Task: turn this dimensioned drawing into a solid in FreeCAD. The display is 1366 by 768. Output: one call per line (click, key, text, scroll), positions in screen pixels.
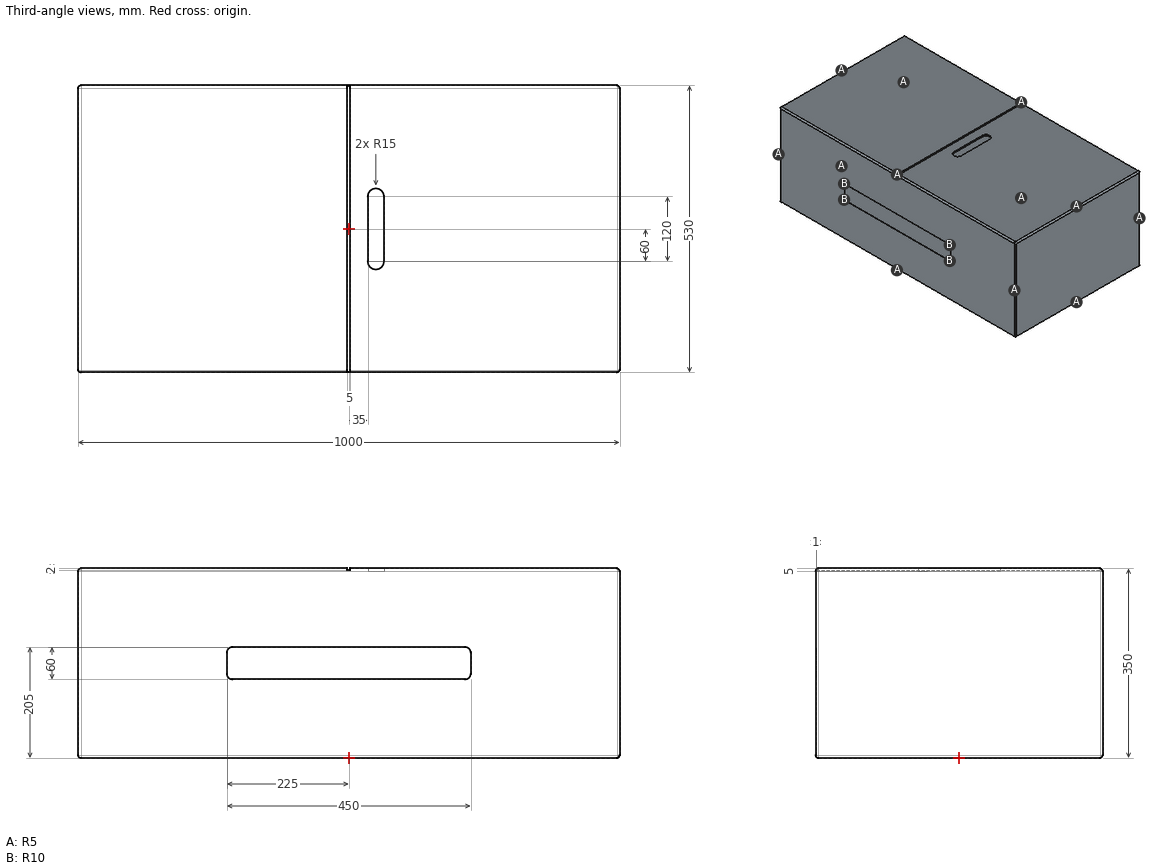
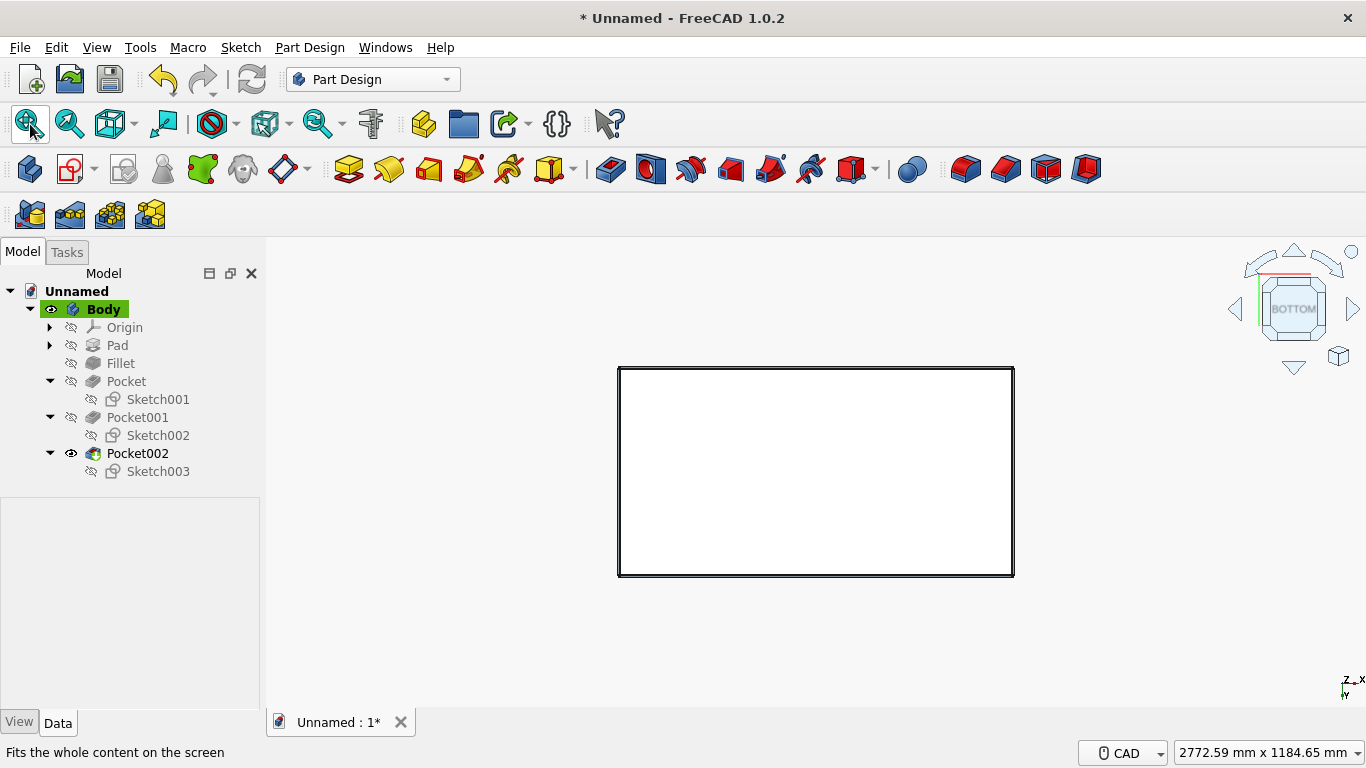
click(30, 124)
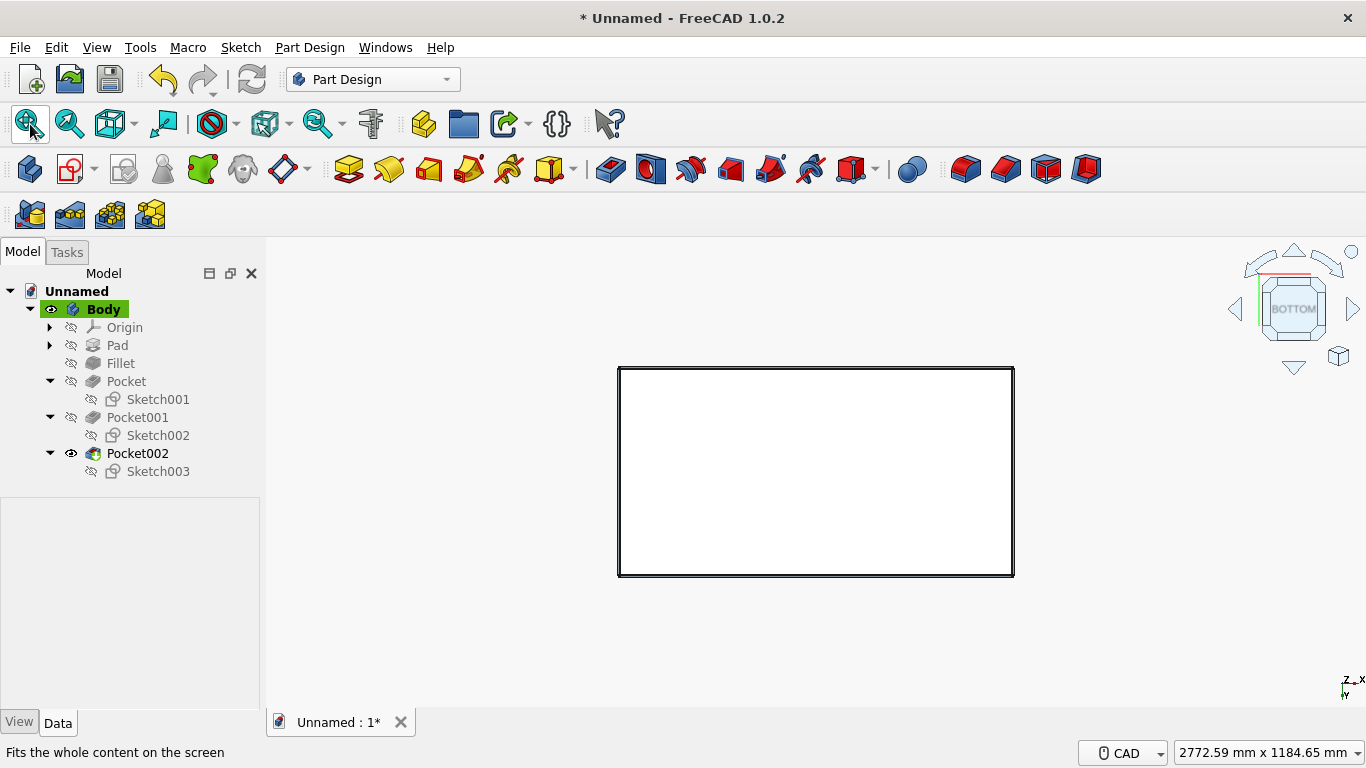
scroll(905, 366, up, 15)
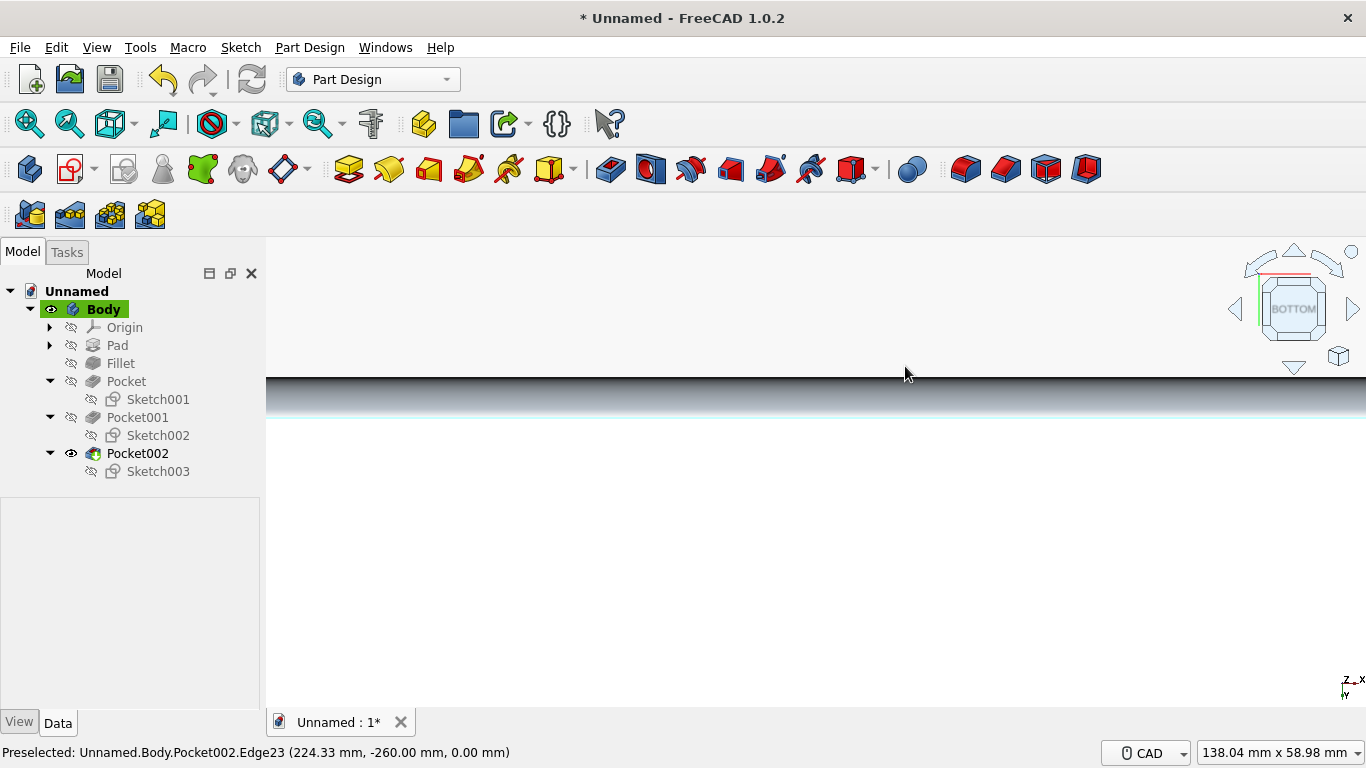
scroll(899, 381, up, 9)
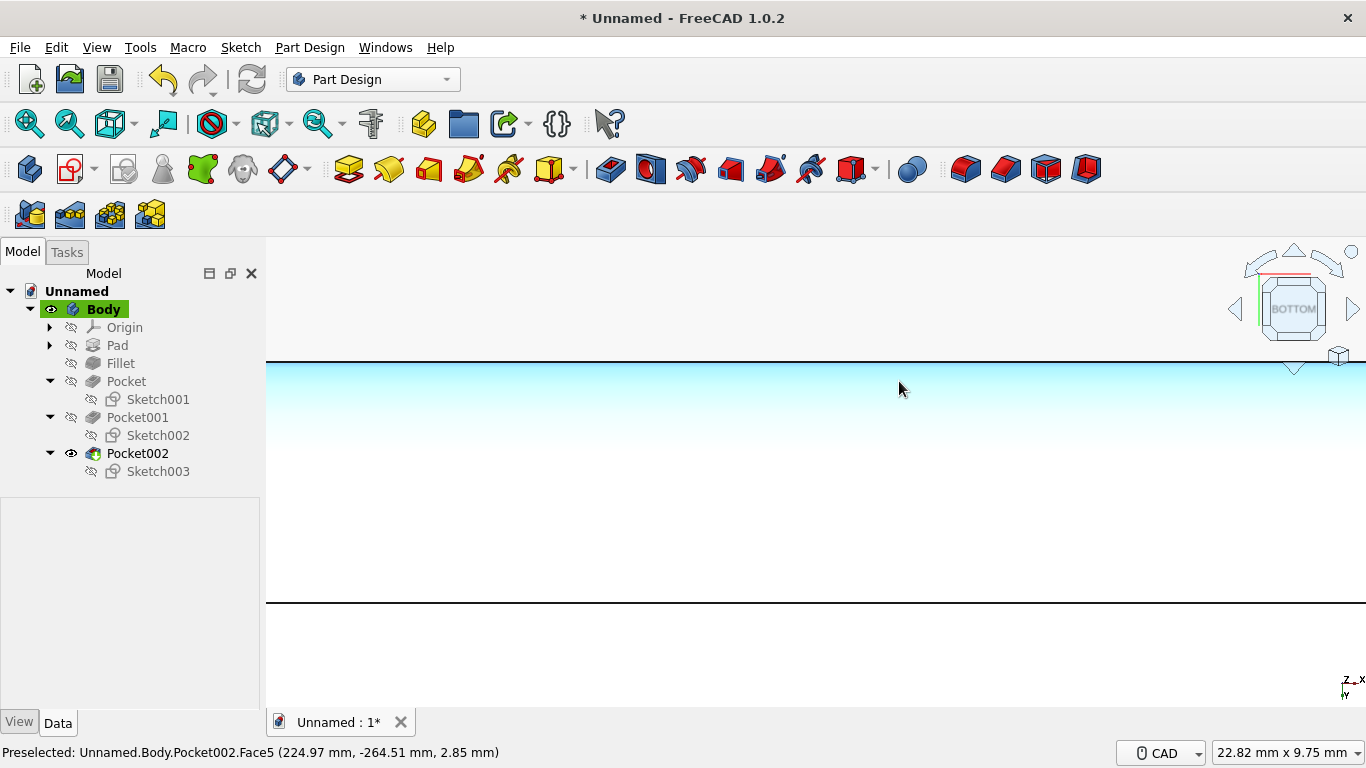
click(30, 124)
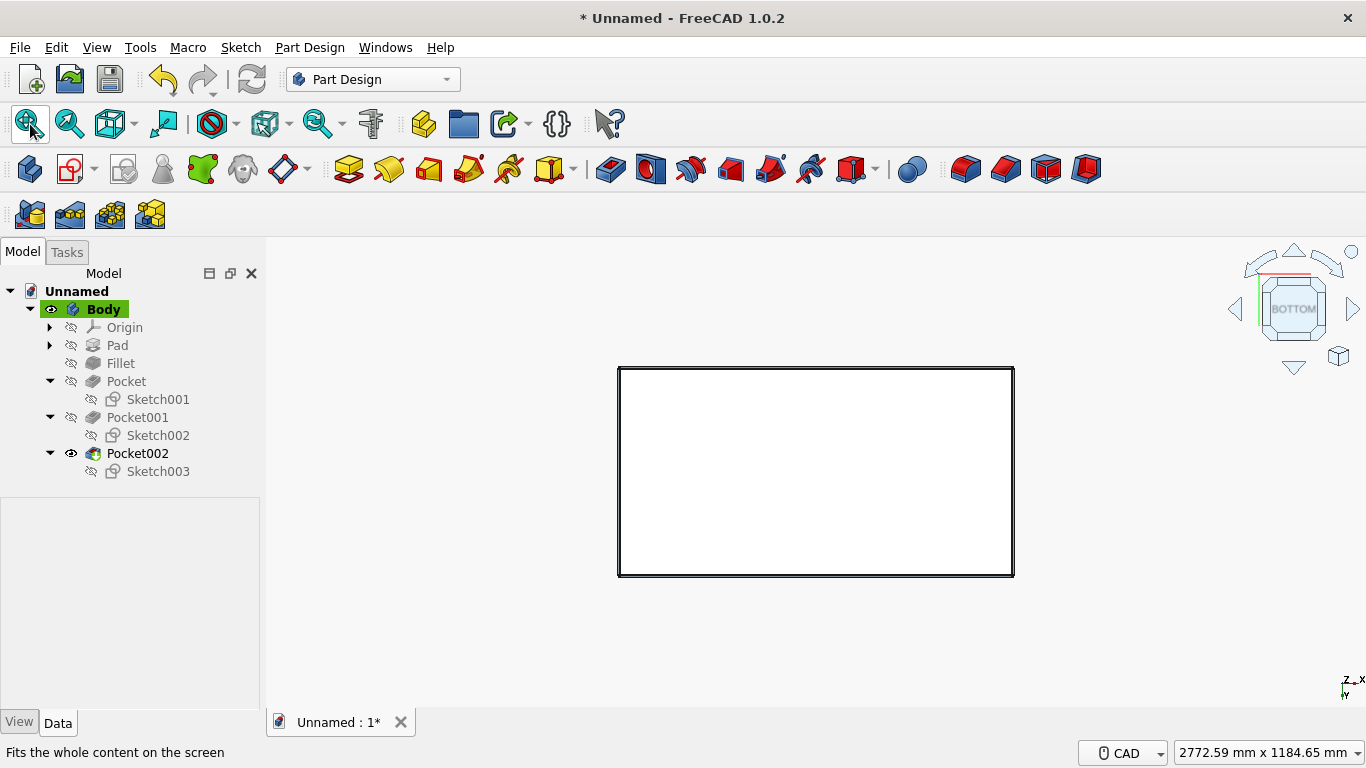
key(4)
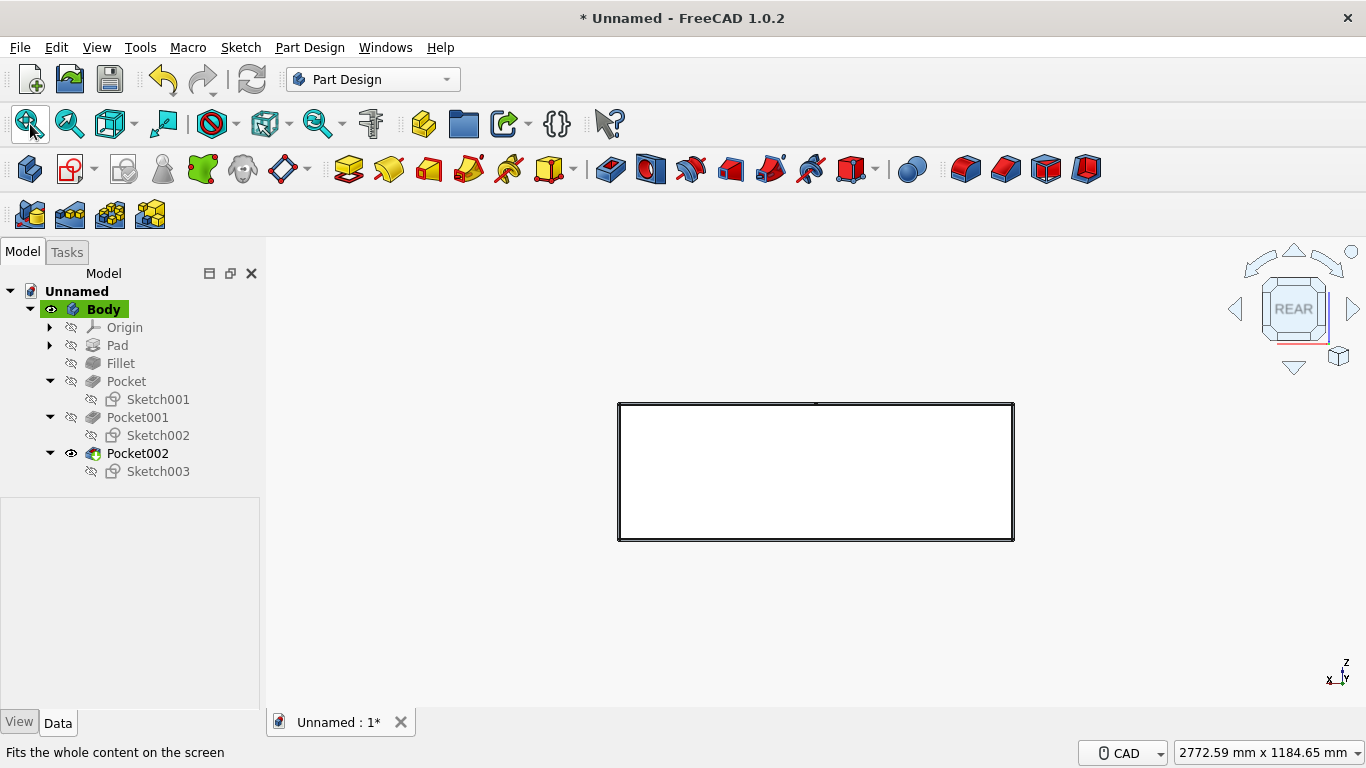
click(30, 124)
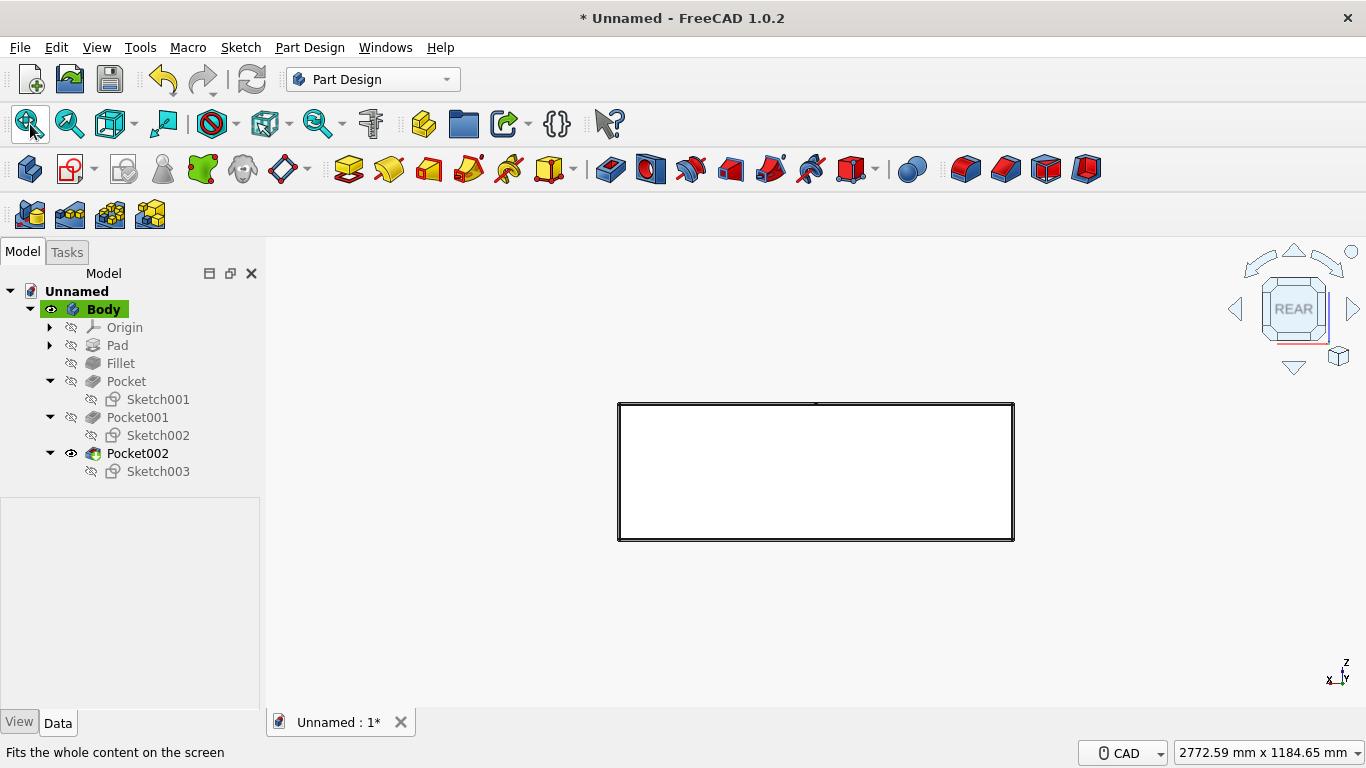
scroll(727, 459, up, 15)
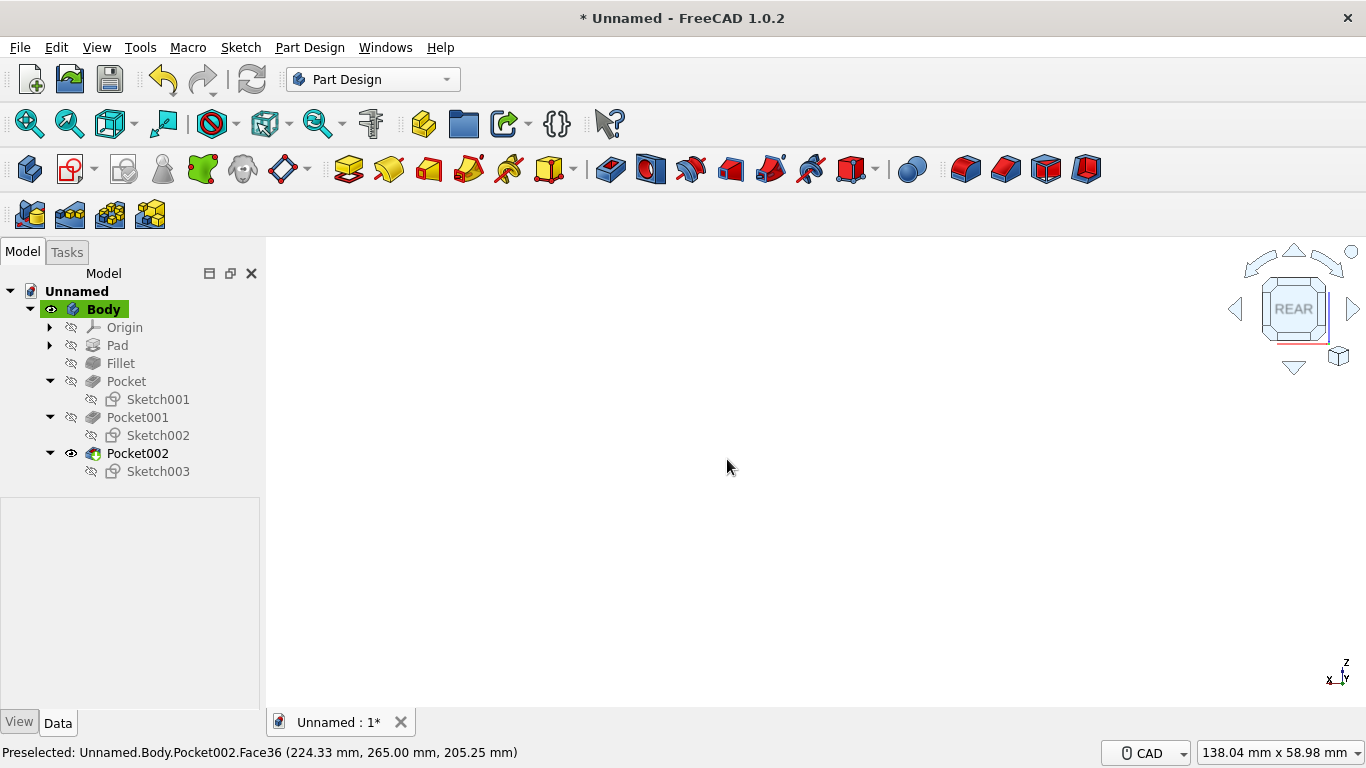
scroll(714, 471, up, 9)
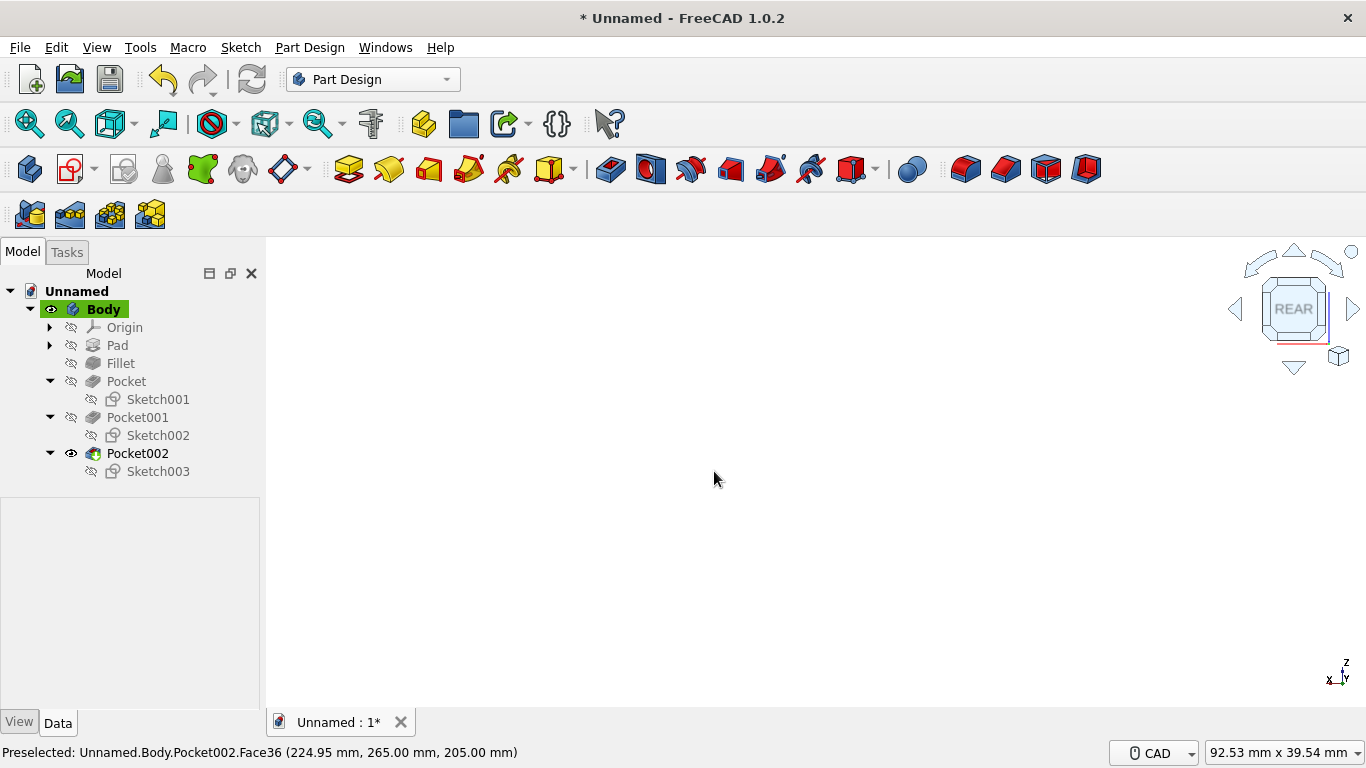
click(30, 124)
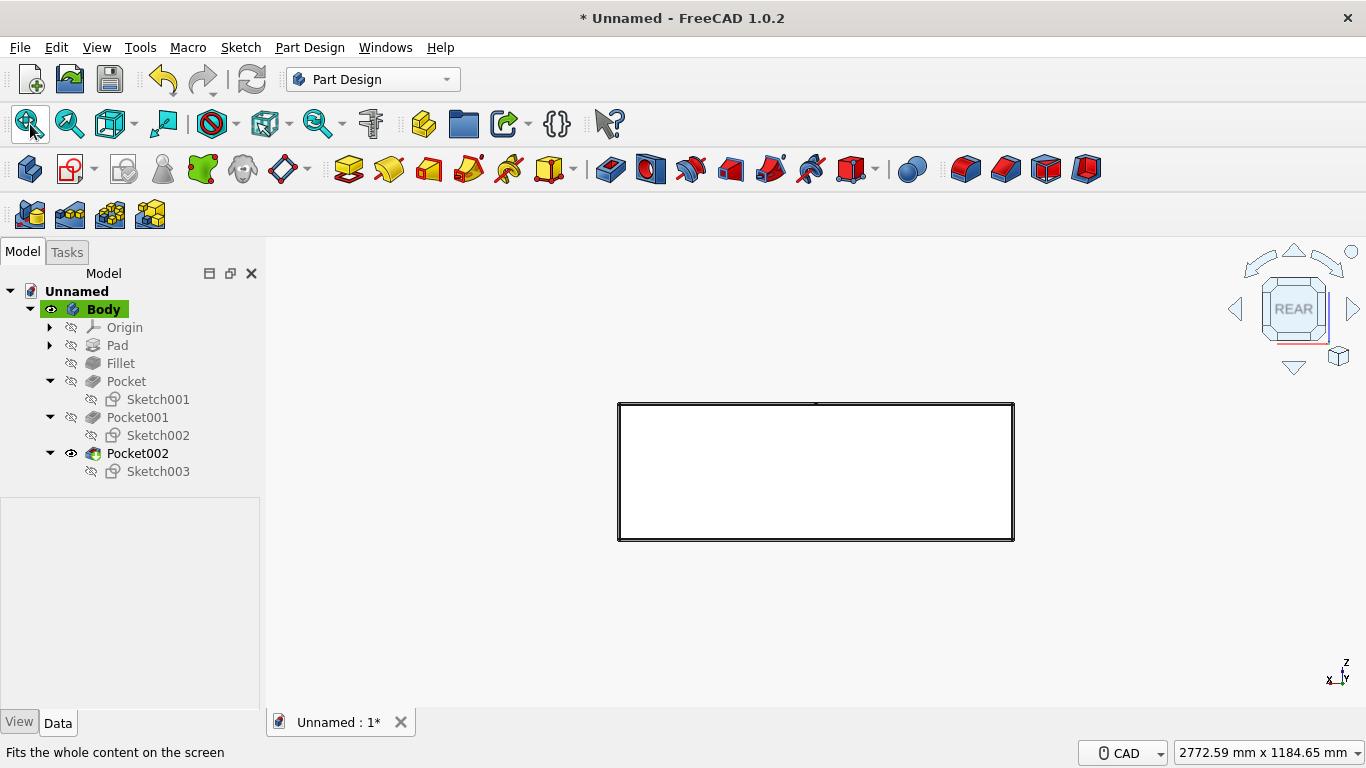
key(6)